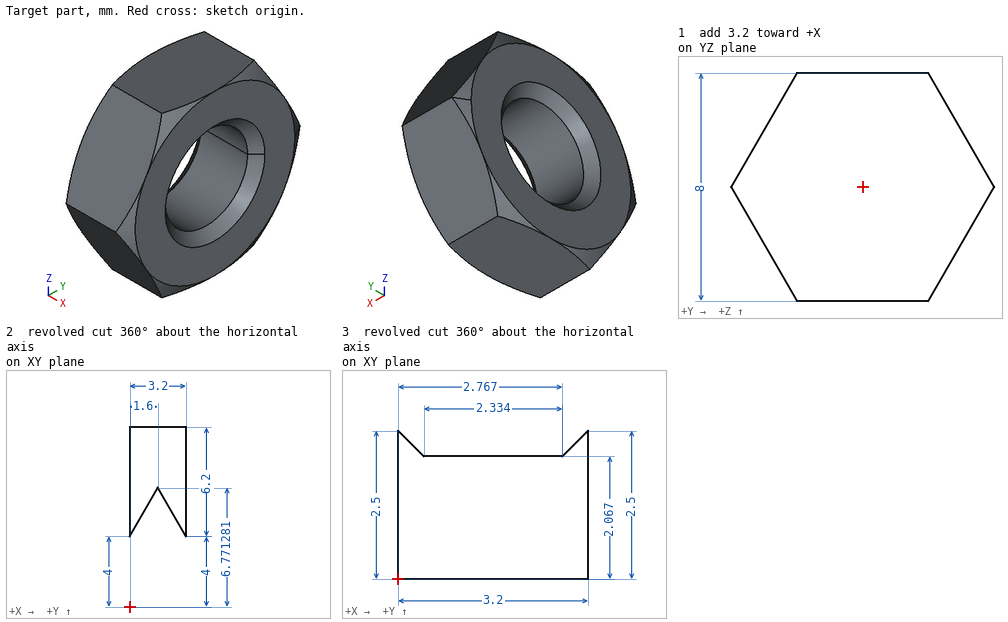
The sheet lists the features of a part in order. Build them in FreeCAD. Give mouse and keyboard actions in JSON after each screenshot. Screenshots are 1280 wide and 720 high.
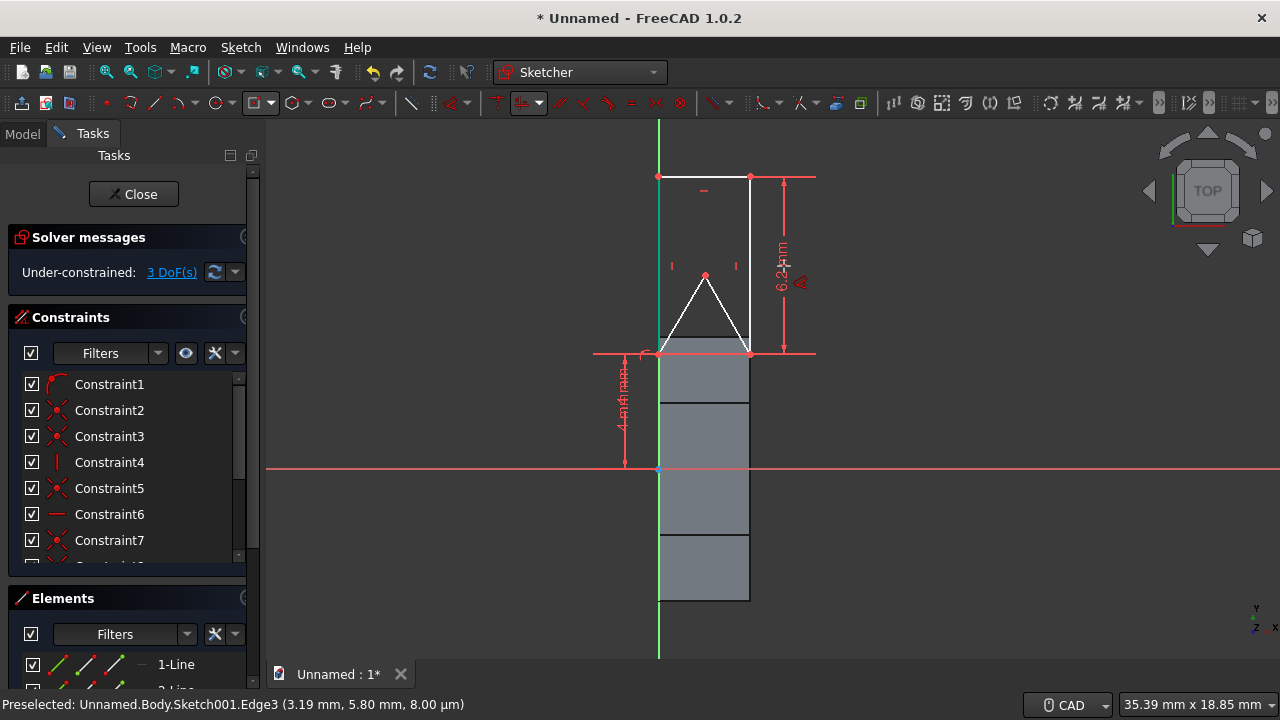
{"action": "left_click", "coordinate": [723, 177]}
{"action": "left_click", "coordinate": [704, 211]}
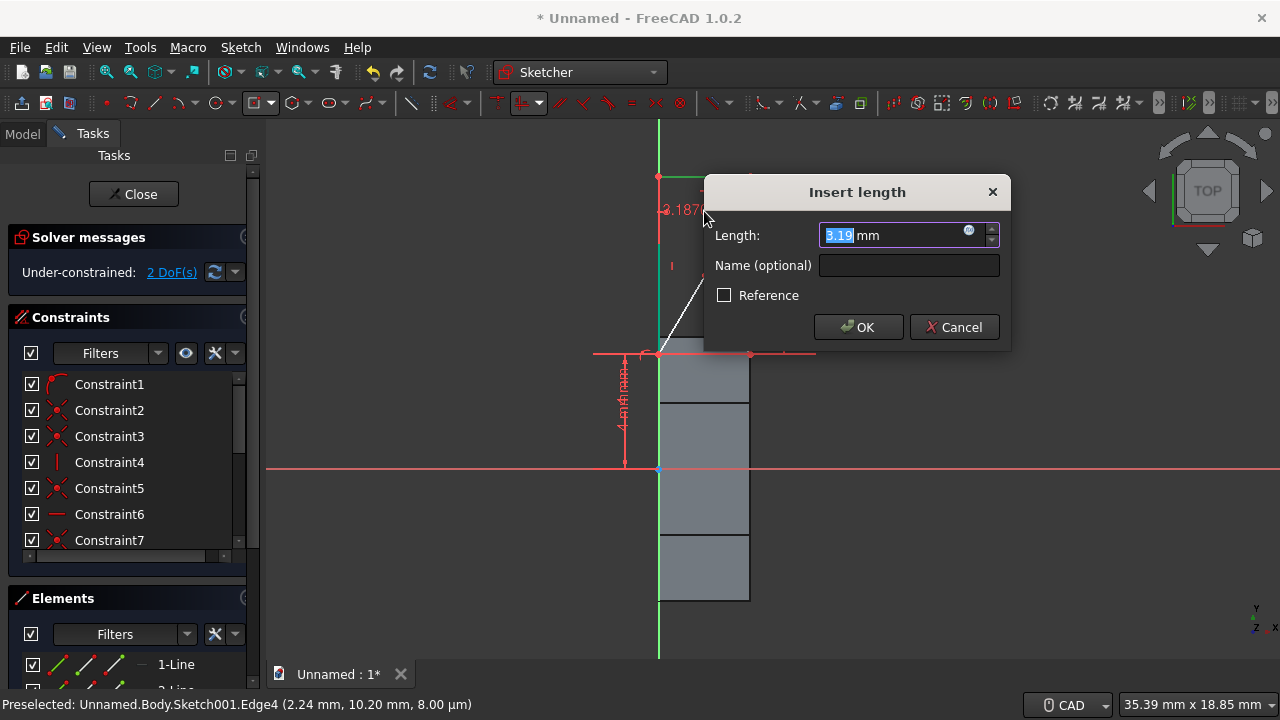
{"action": "type", "text": "3.2"}
{"action": "key", "text": "Return"}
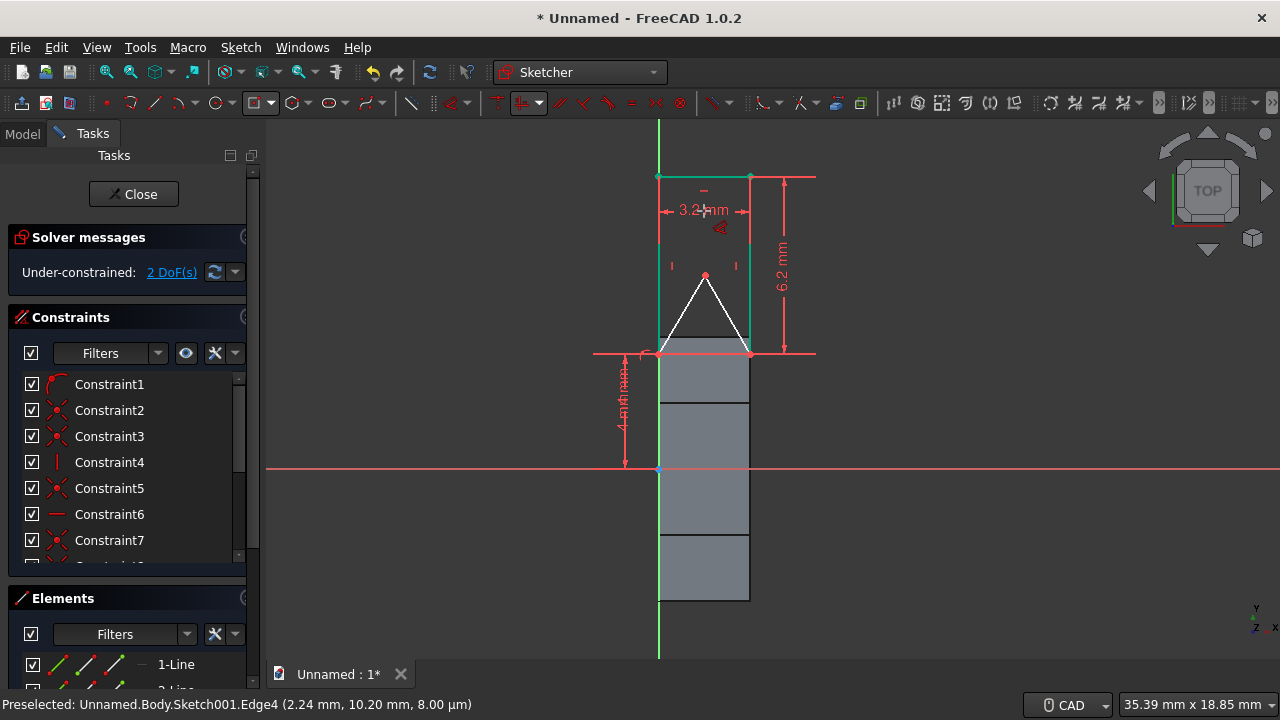
{"action": "left_click", "coordinate": [705, 276]}
{"action": "left_click", "coordinate": [682, 503]}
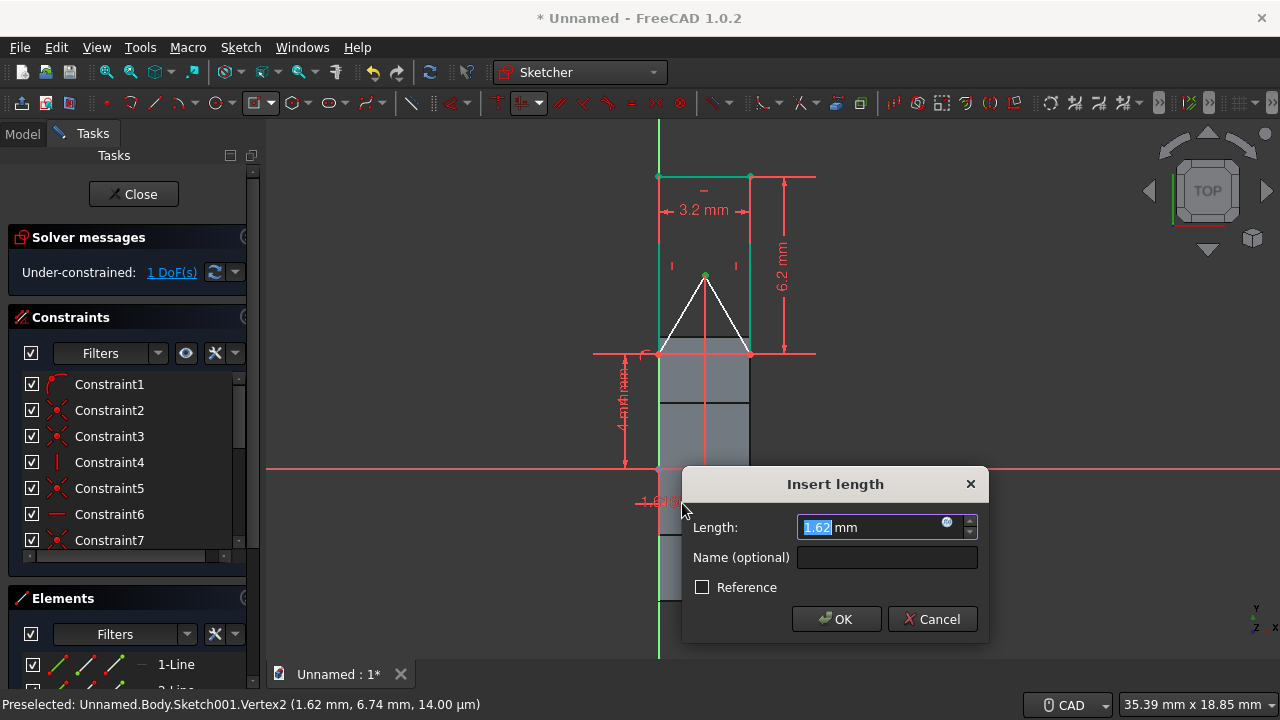
{"action": "type", "text": "1.6"}
{"action": "key", "text": "Return"}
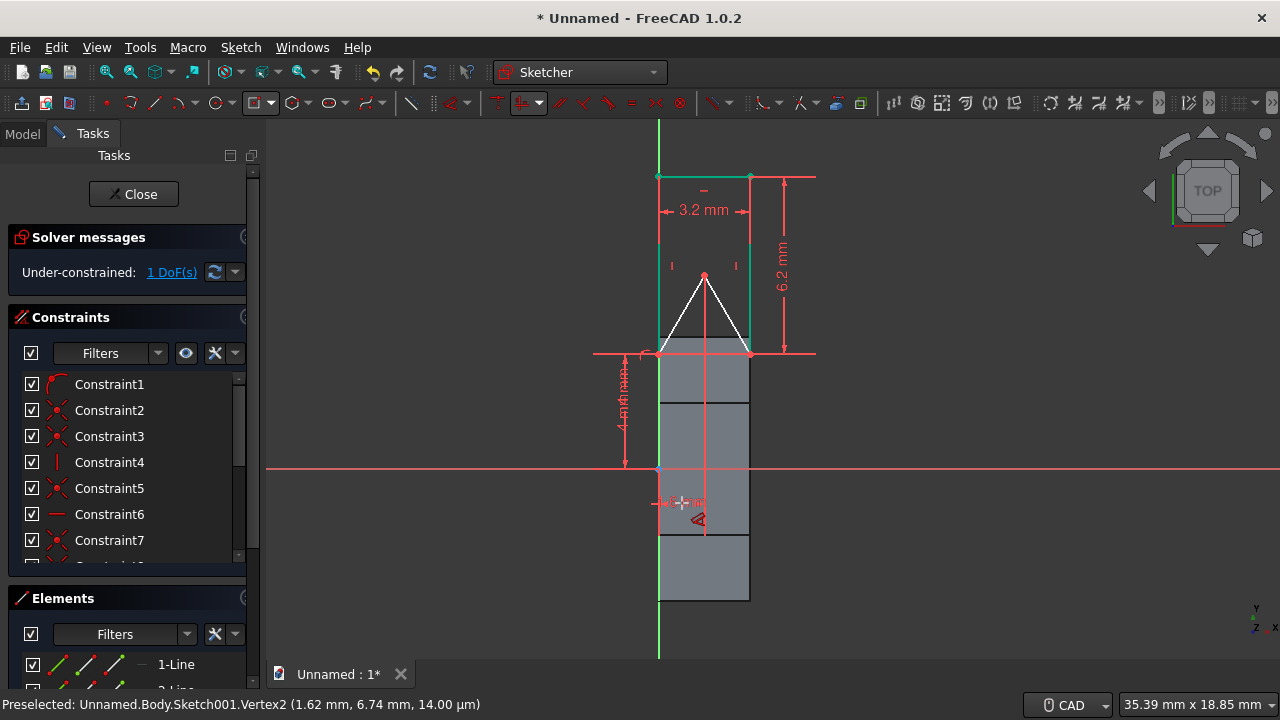
{"action": "left_click", "coordinate": [705, 276]}
{"action": "left_click", "coordinate": [625, 328]}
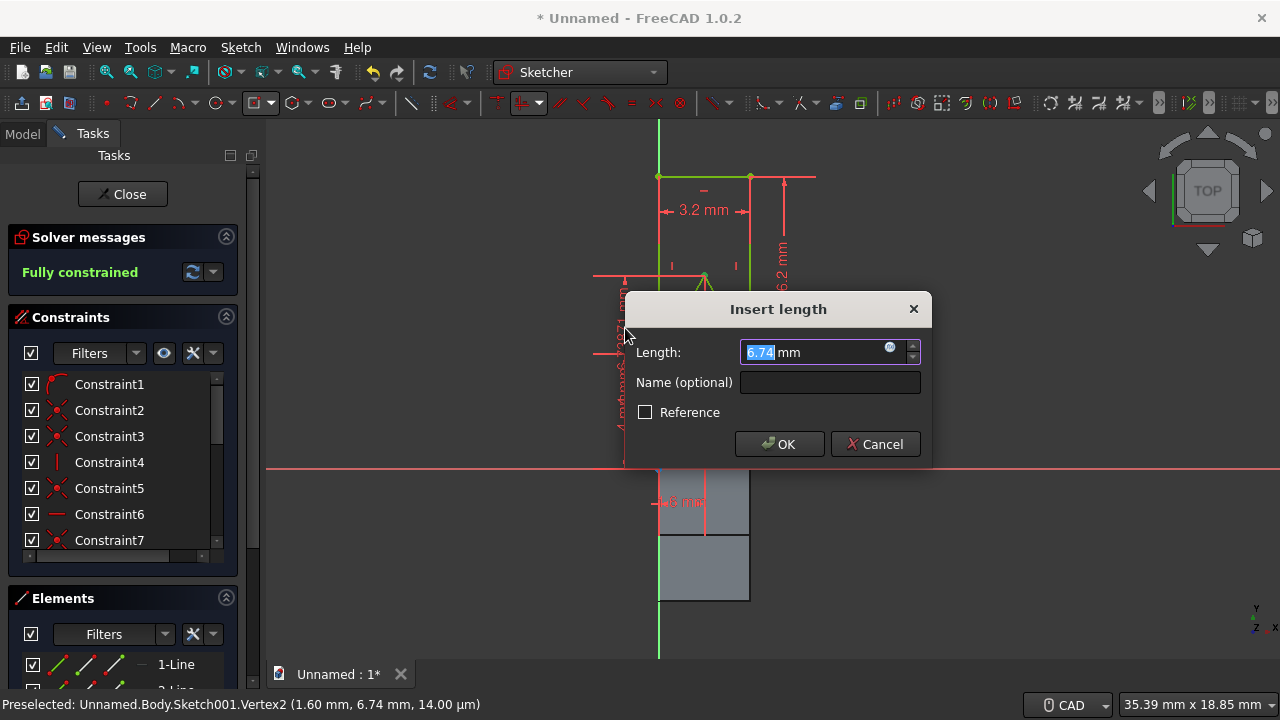
{"action": "type", "text": "6.771281"}
{"action": "key", "text": "Return"}
{"action": "key", "text": "Escape"}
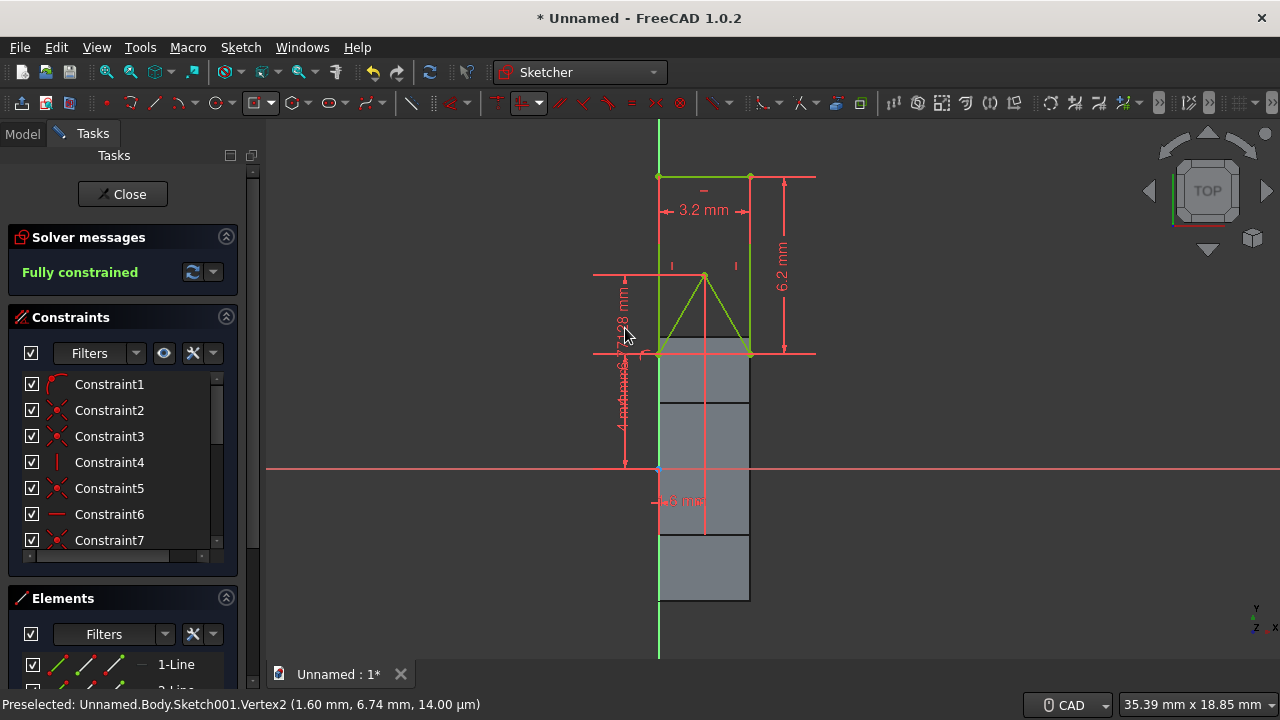
{"action": "left_click", "coordinate": [123, 194]}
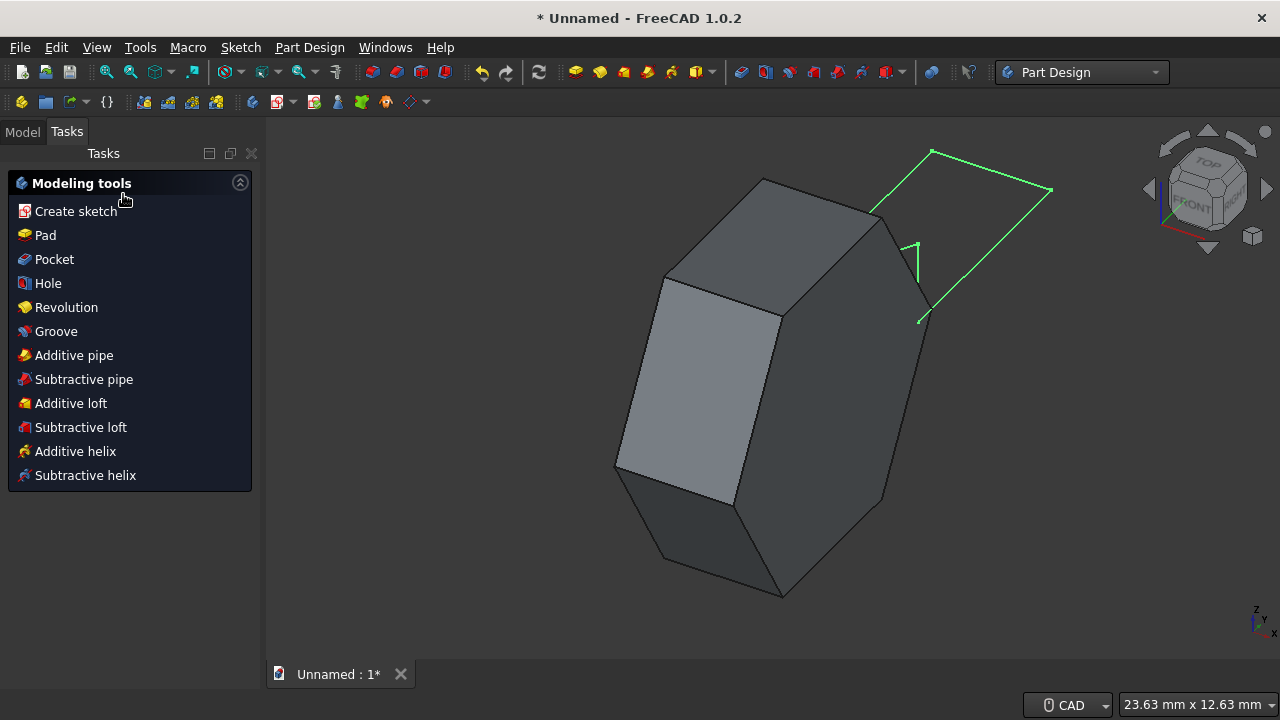
{"action": "left_click", "coordinate": [790, 72]}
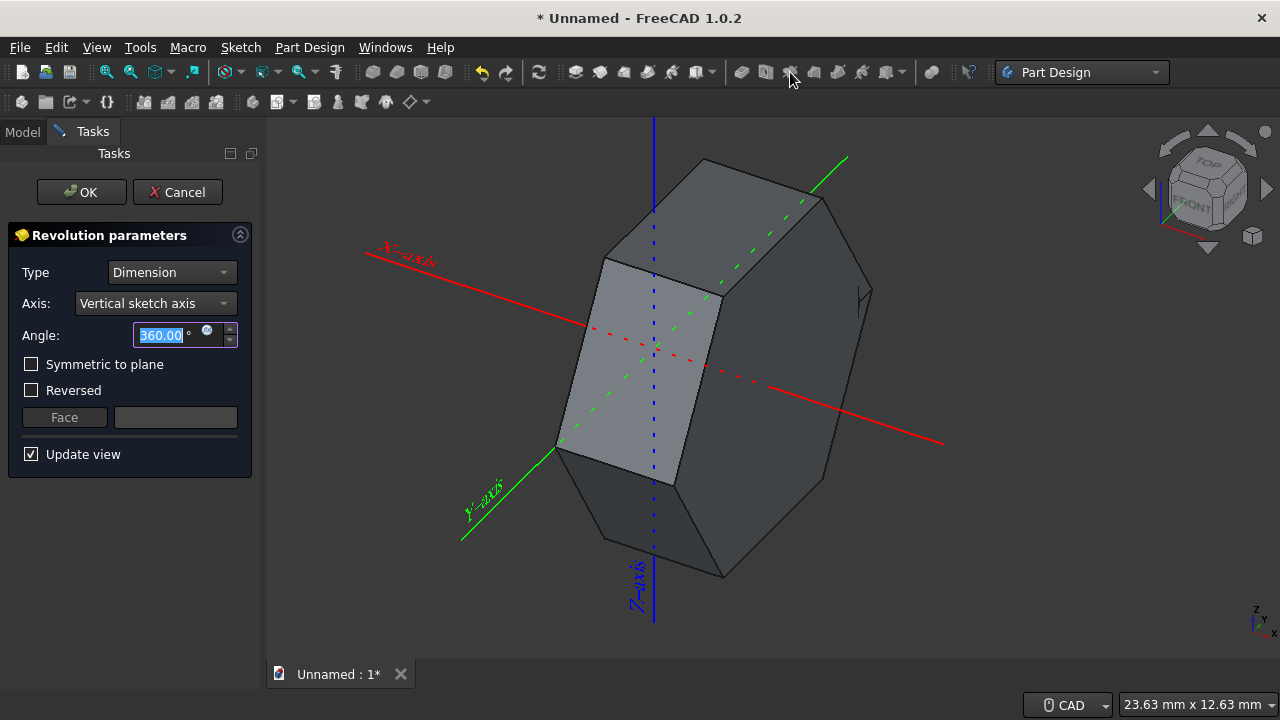
{"action": "left_click", "coordinate": [156, 304]}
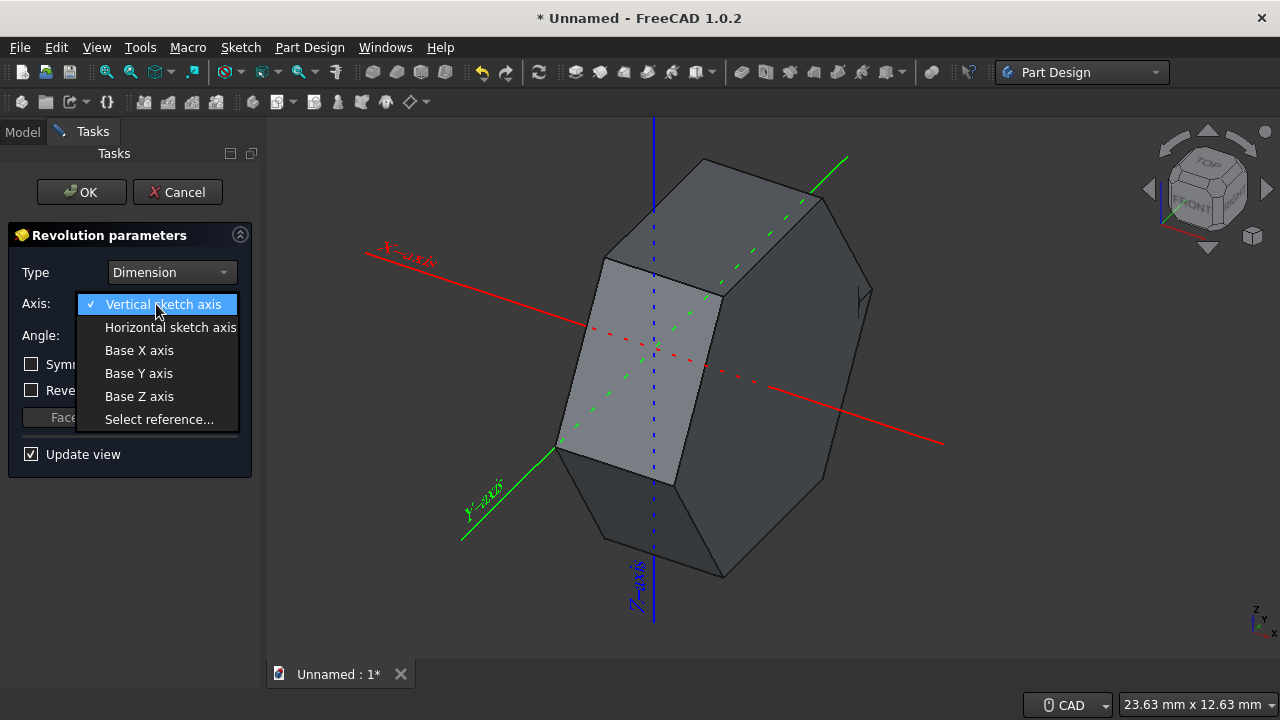
{"action": "left_click", "coordinate": [156, 328]}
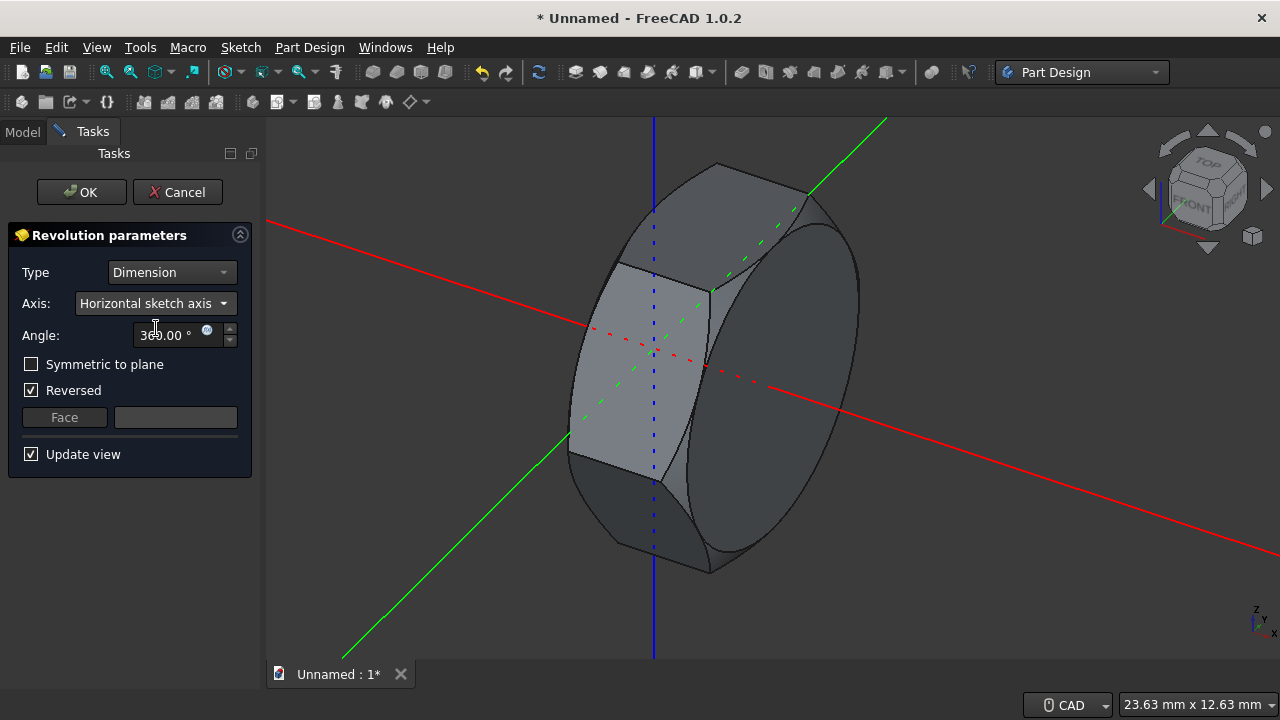
{"action": "left_click", "coordinate": [82, 192]}